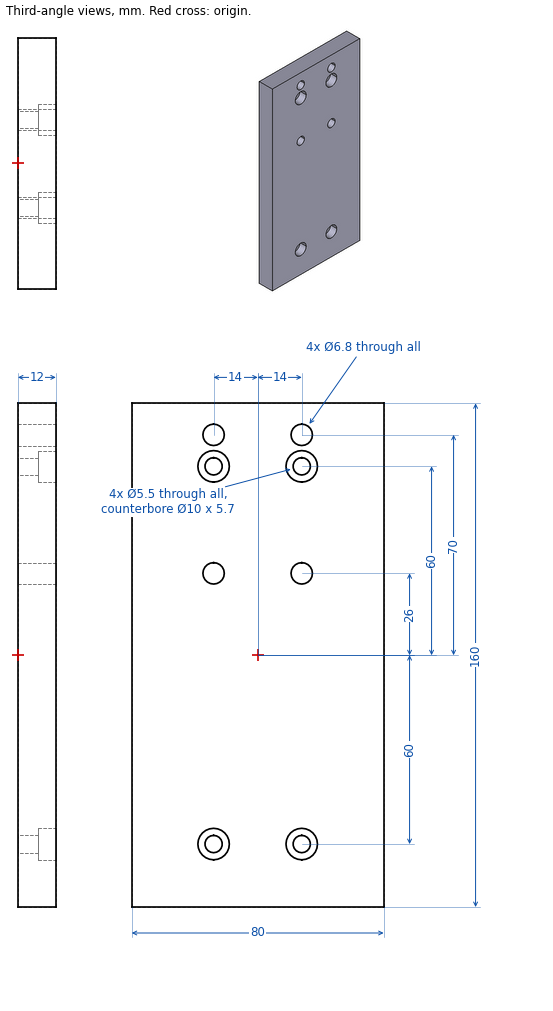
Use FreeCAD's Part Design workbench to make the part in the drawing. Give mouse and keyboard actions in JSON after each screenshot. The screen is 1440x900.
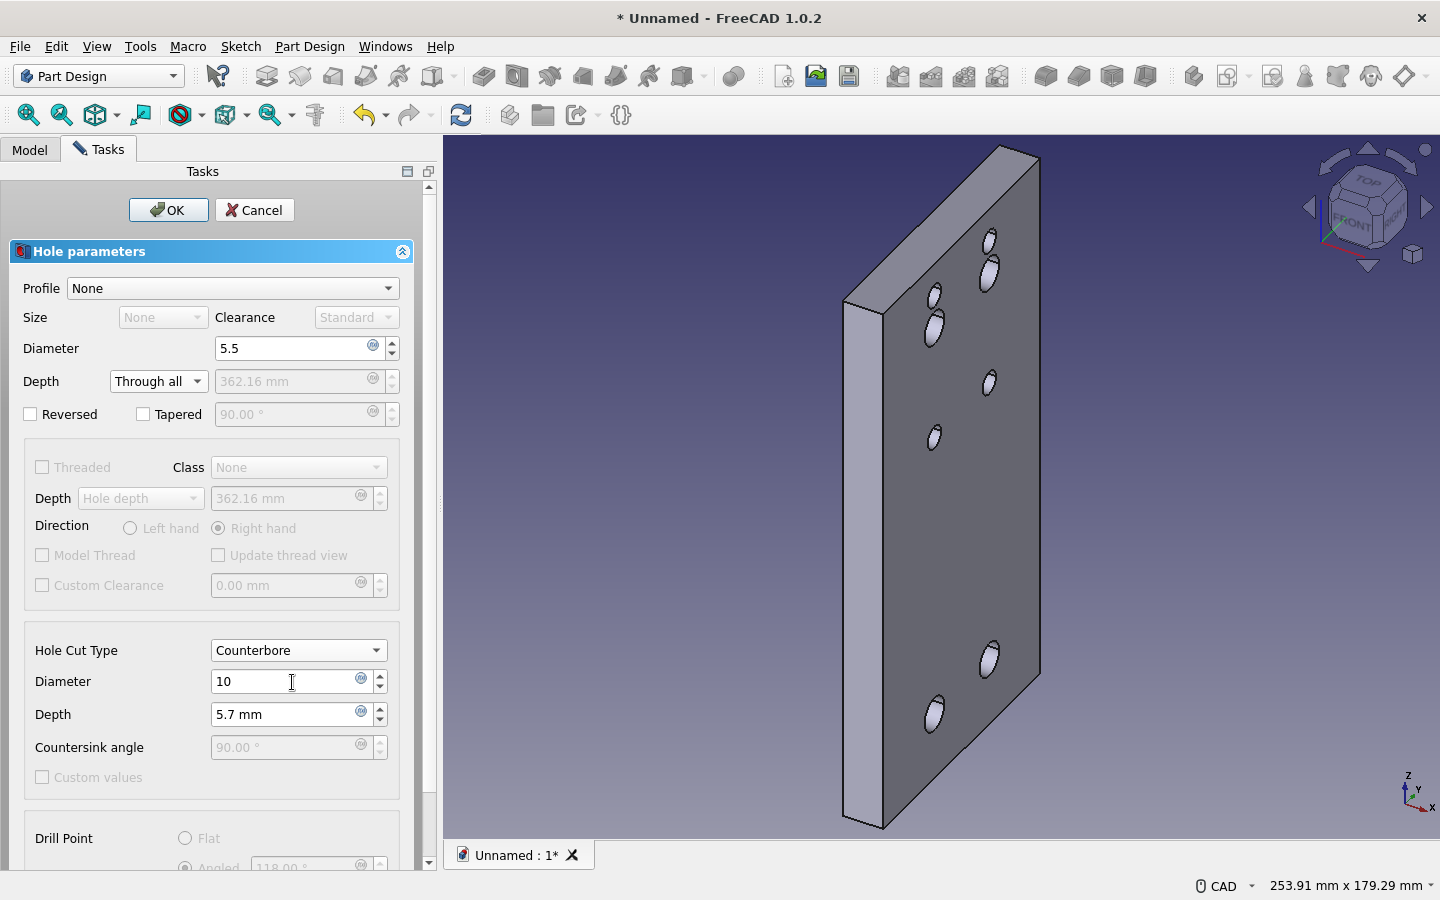
{"action": "left_click", "coordinate": [169, 210]}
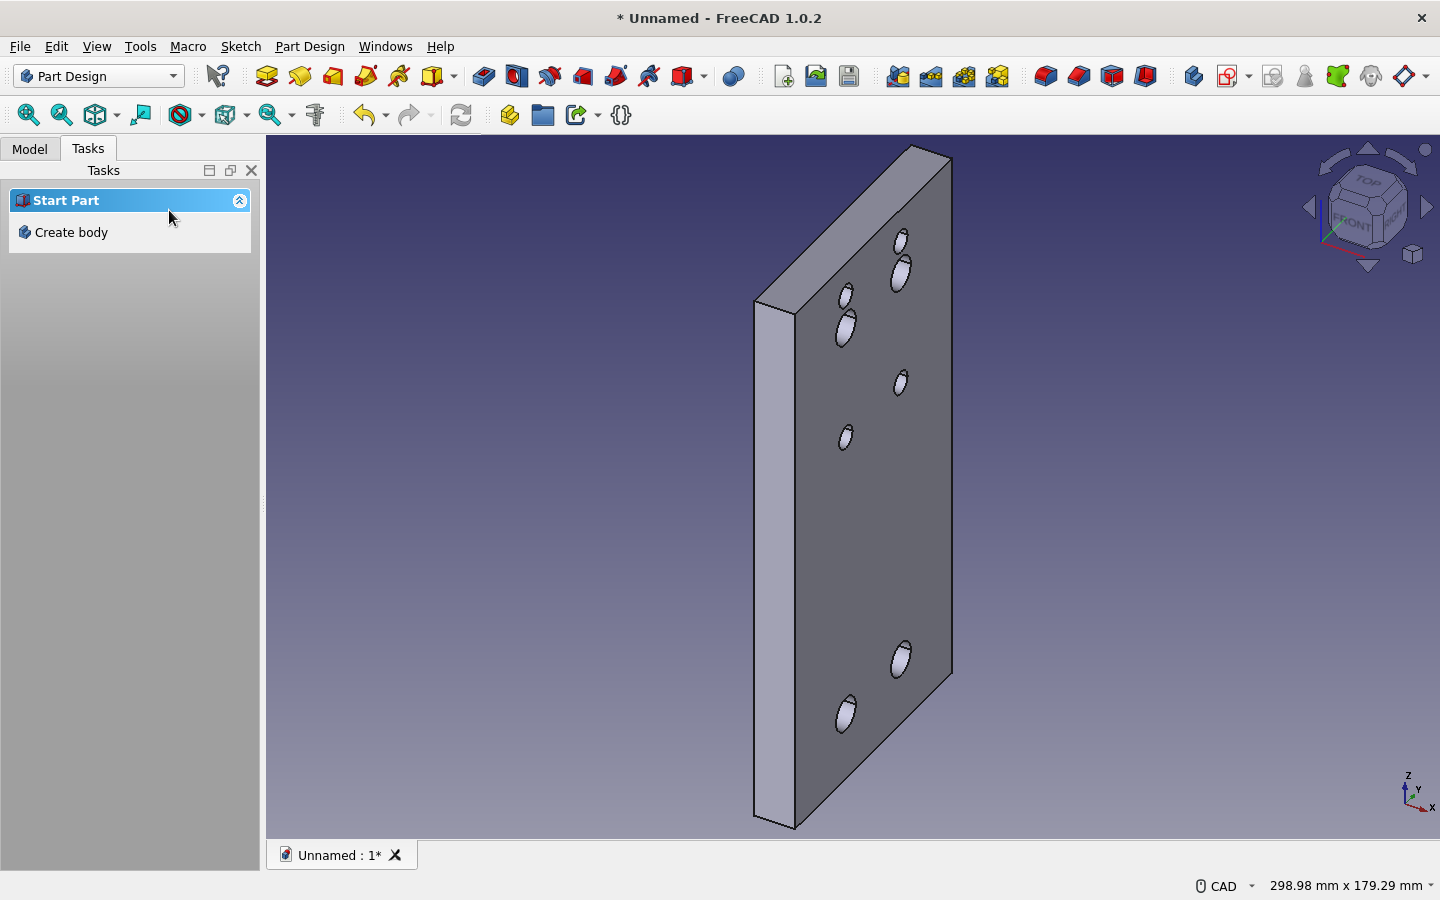
{"action": "key", "text": "0"}